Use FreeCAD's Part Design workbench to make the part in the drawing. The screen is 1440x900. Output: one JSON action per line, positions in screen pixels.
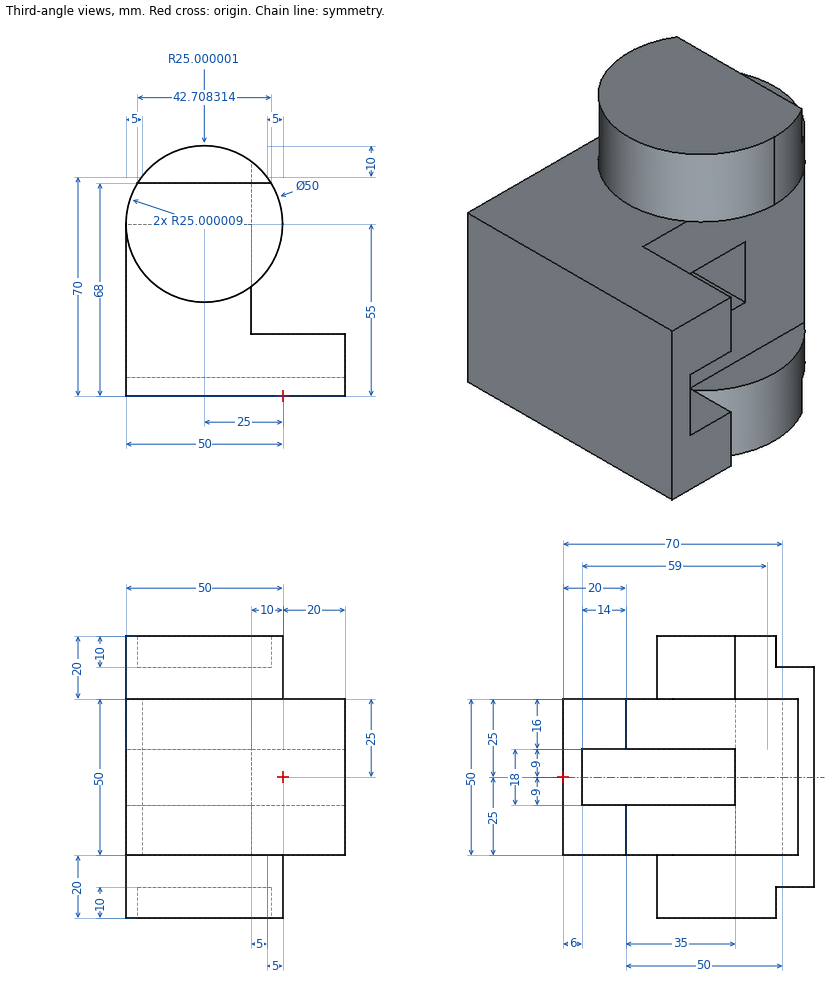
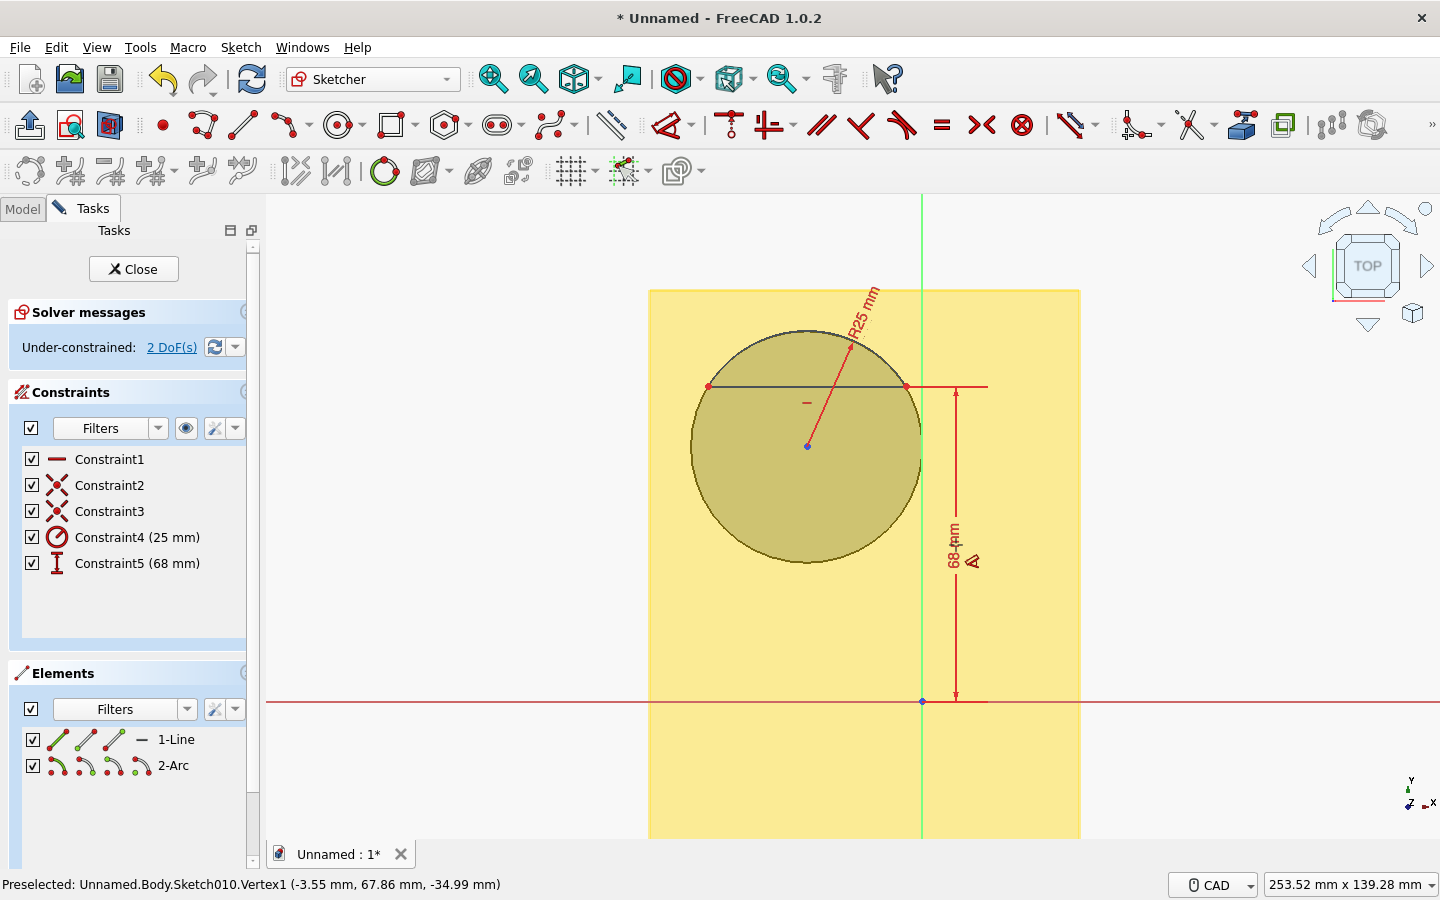
{"action": "left_click", "coordinate": [807, 447]}
{"action": "left_click", "coordinate": [865, 736]}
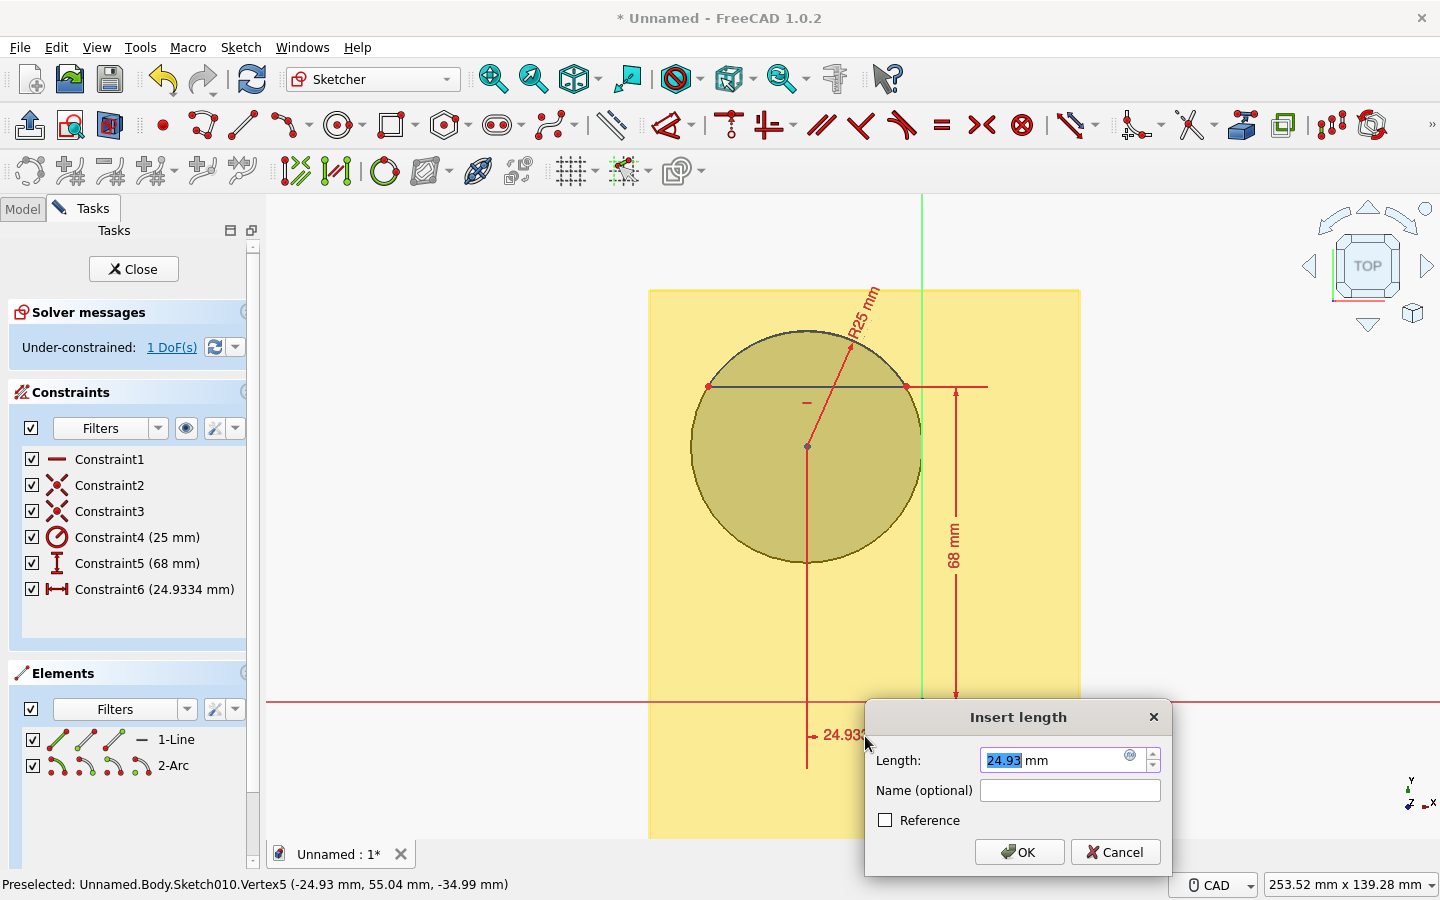
{"action": "type", "text": "25"}
{"action": "key", "text": "Return"}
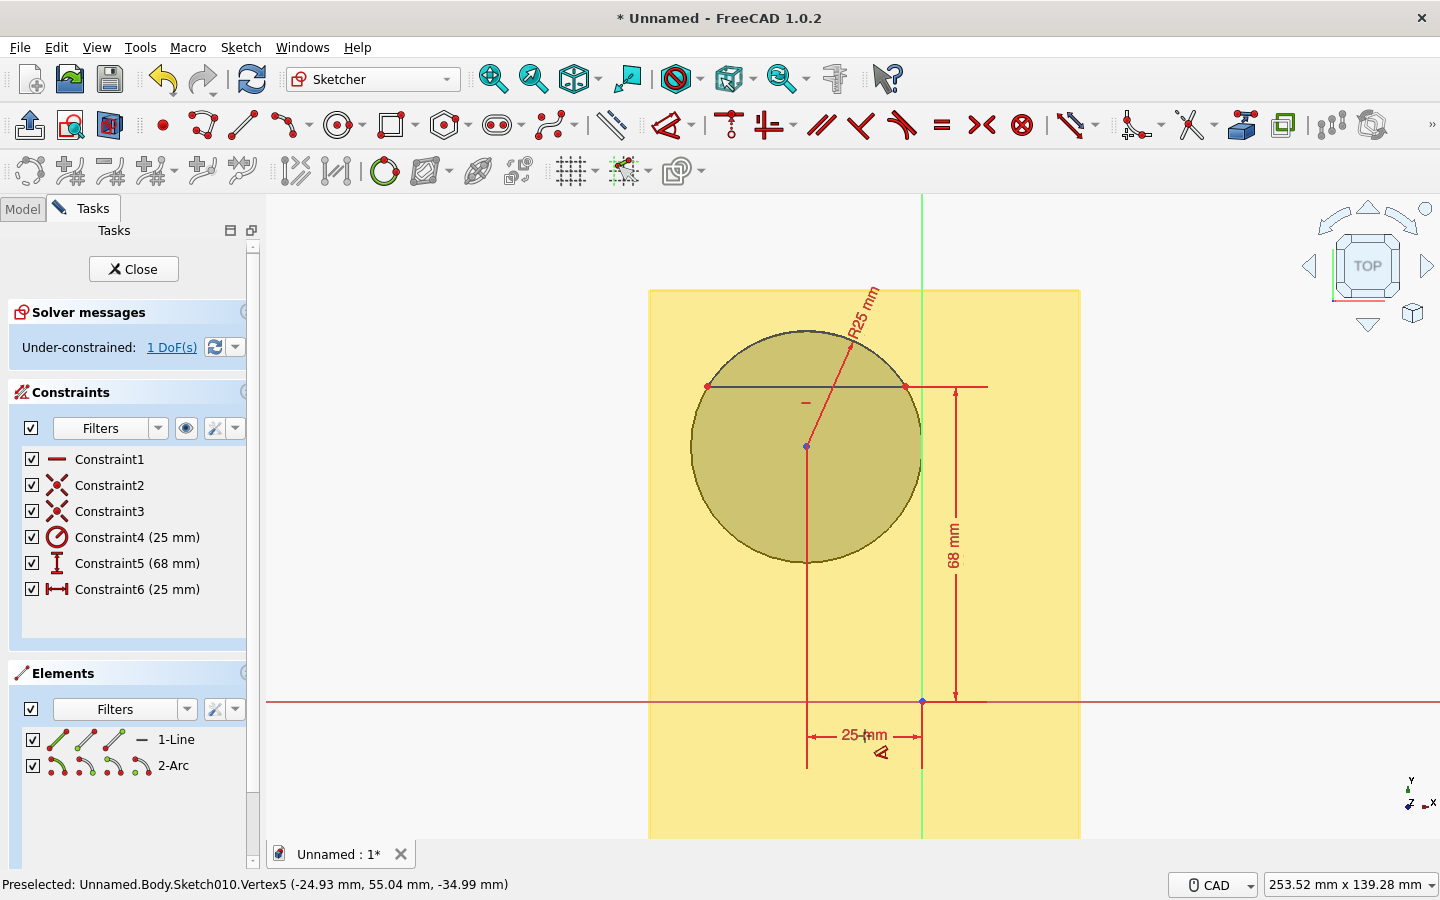
{"action": "left_click", "coordinate": [846, 387]}
{"action": "left_click", "coordinate": [807, 353]}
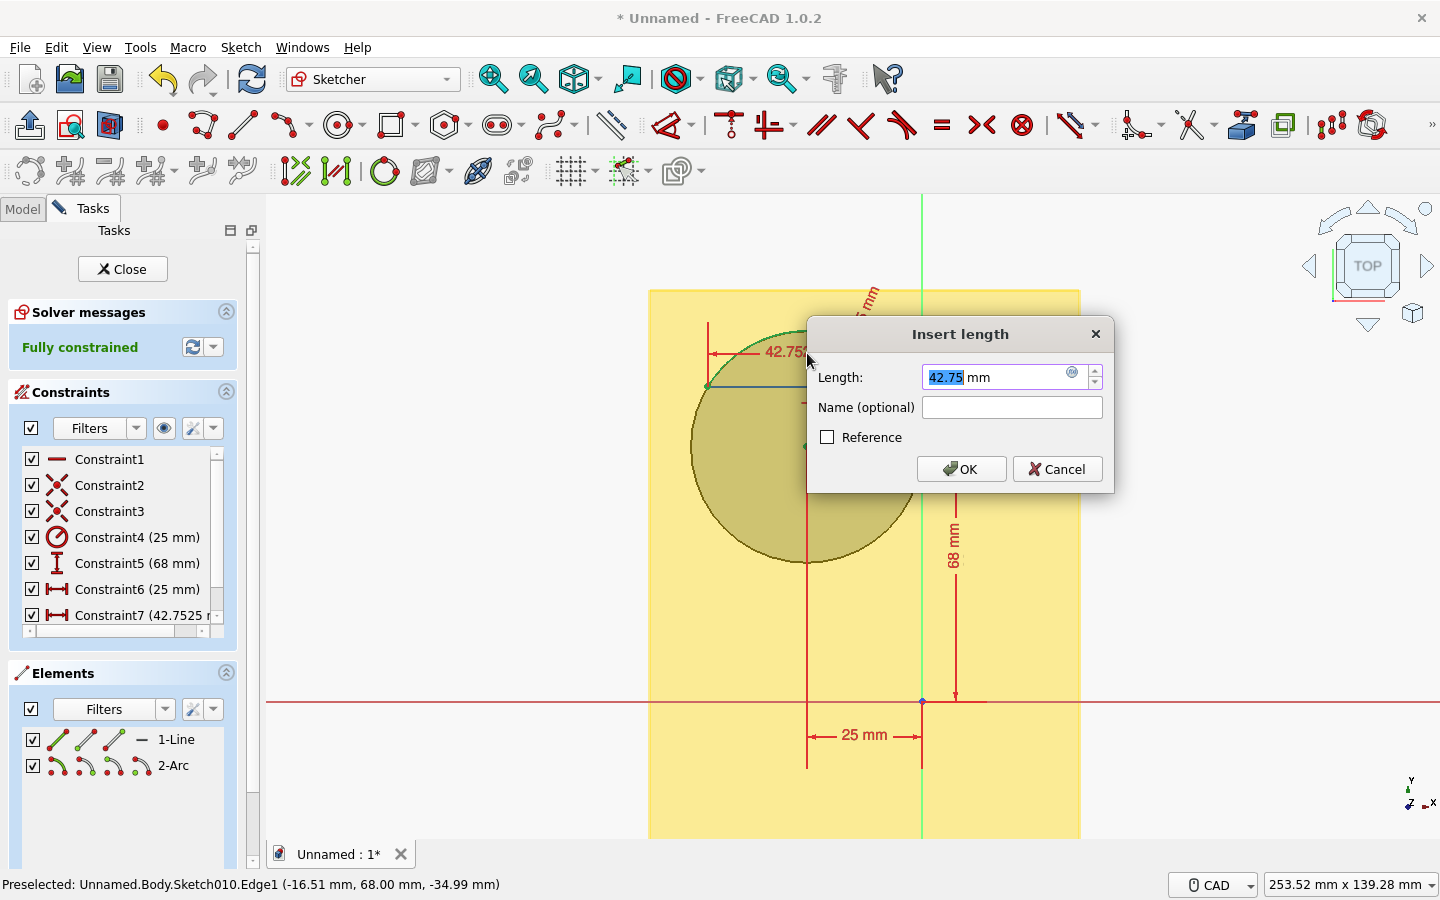
{"action": "type", "text": "42.708314"}
{"action": "key", "text": "Return"}
{"action": "key", "text": "Escape"}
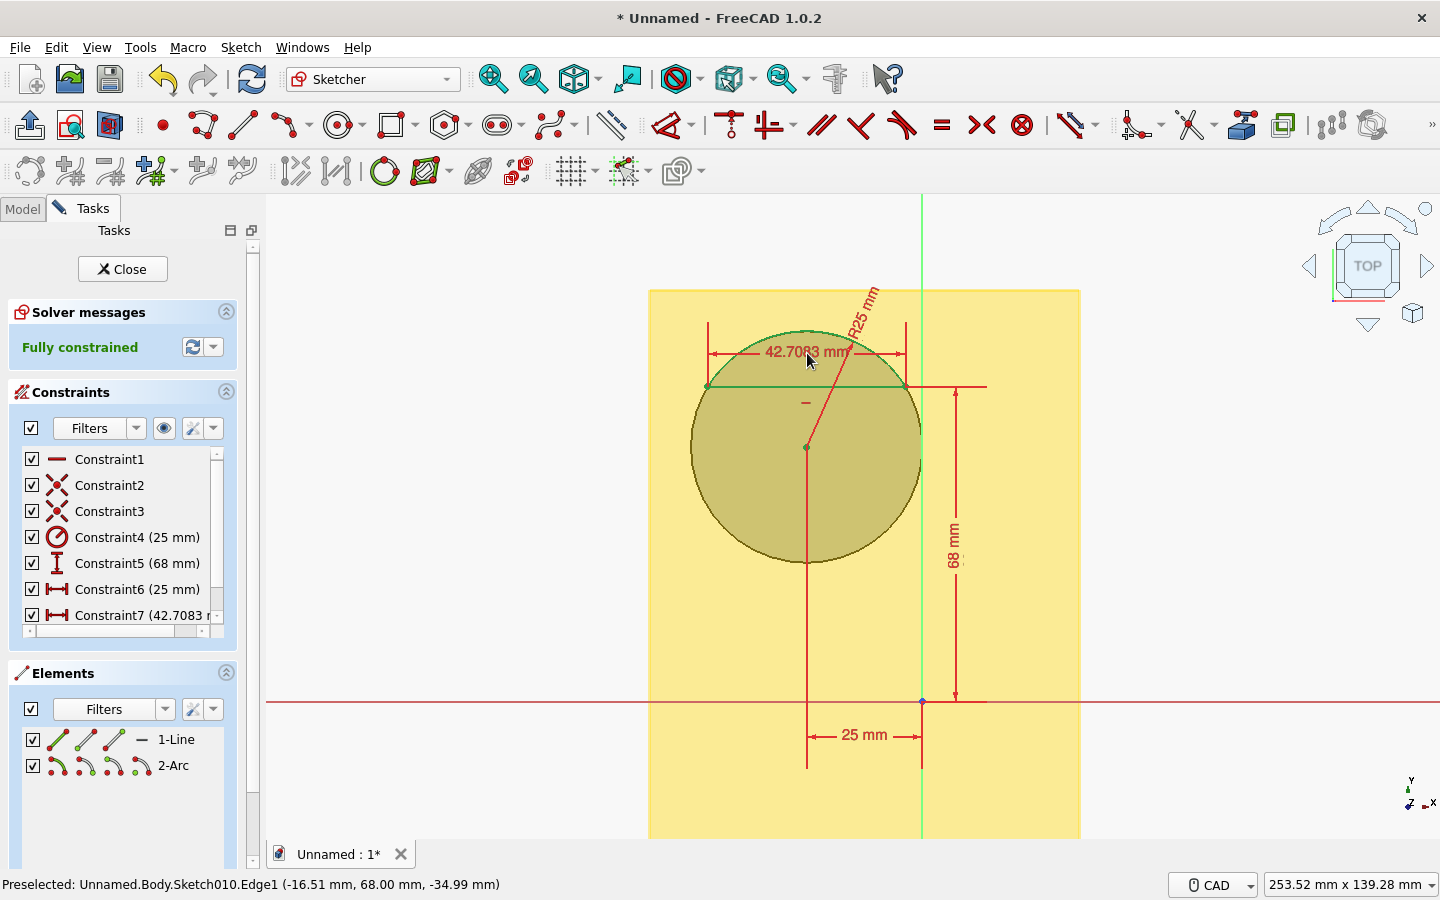
{"action": "left_click", "coordinate": [123, 269]}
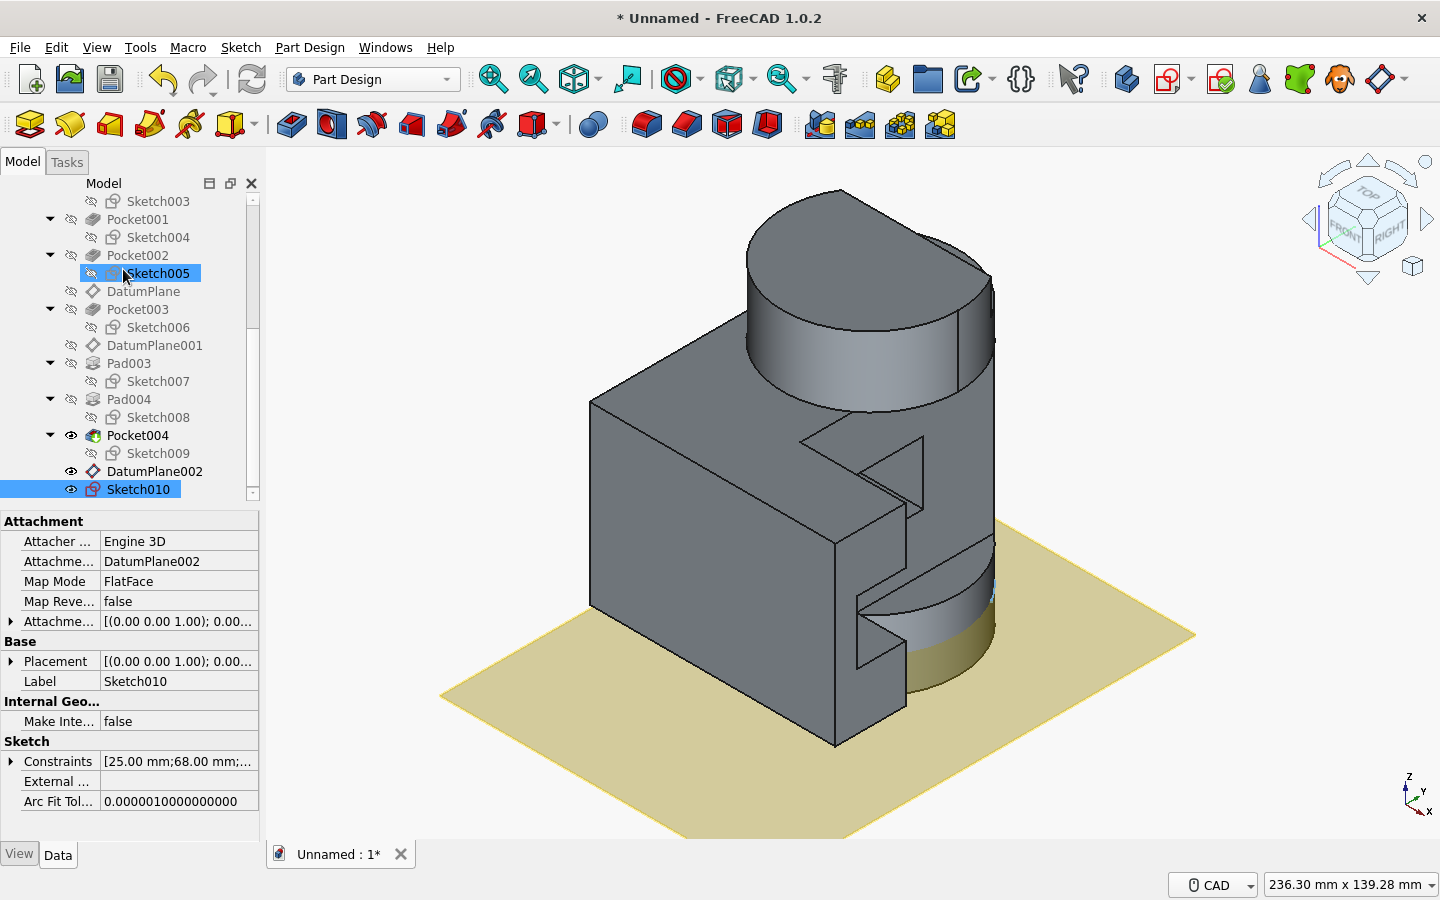
{"action": "left_click", "coordinate": [292, 124]}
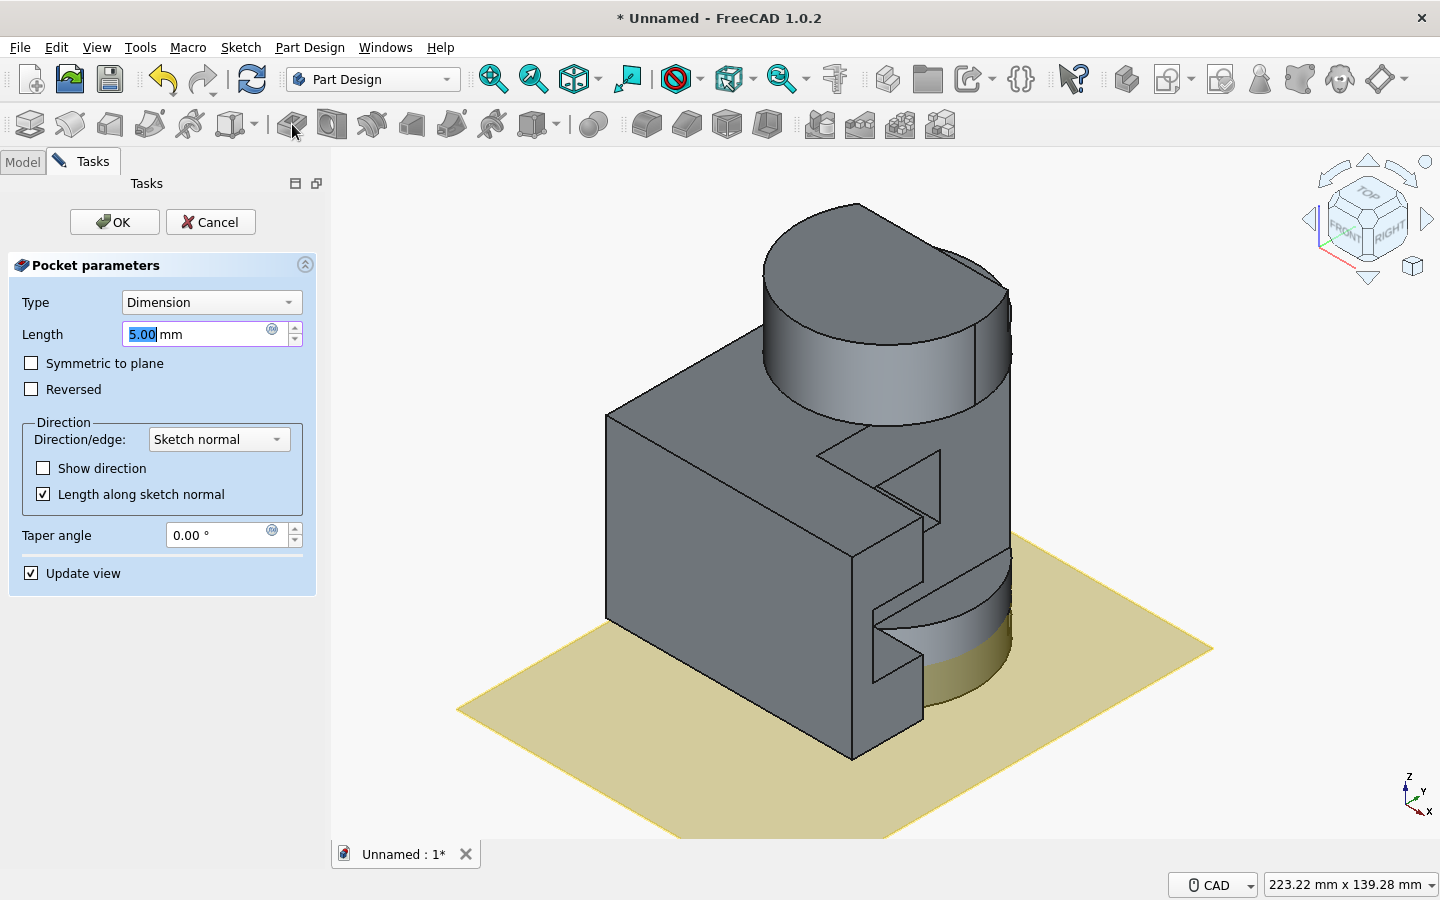
{"action": "type", "text": "10"}
{"action": "key", "text": "Tab"}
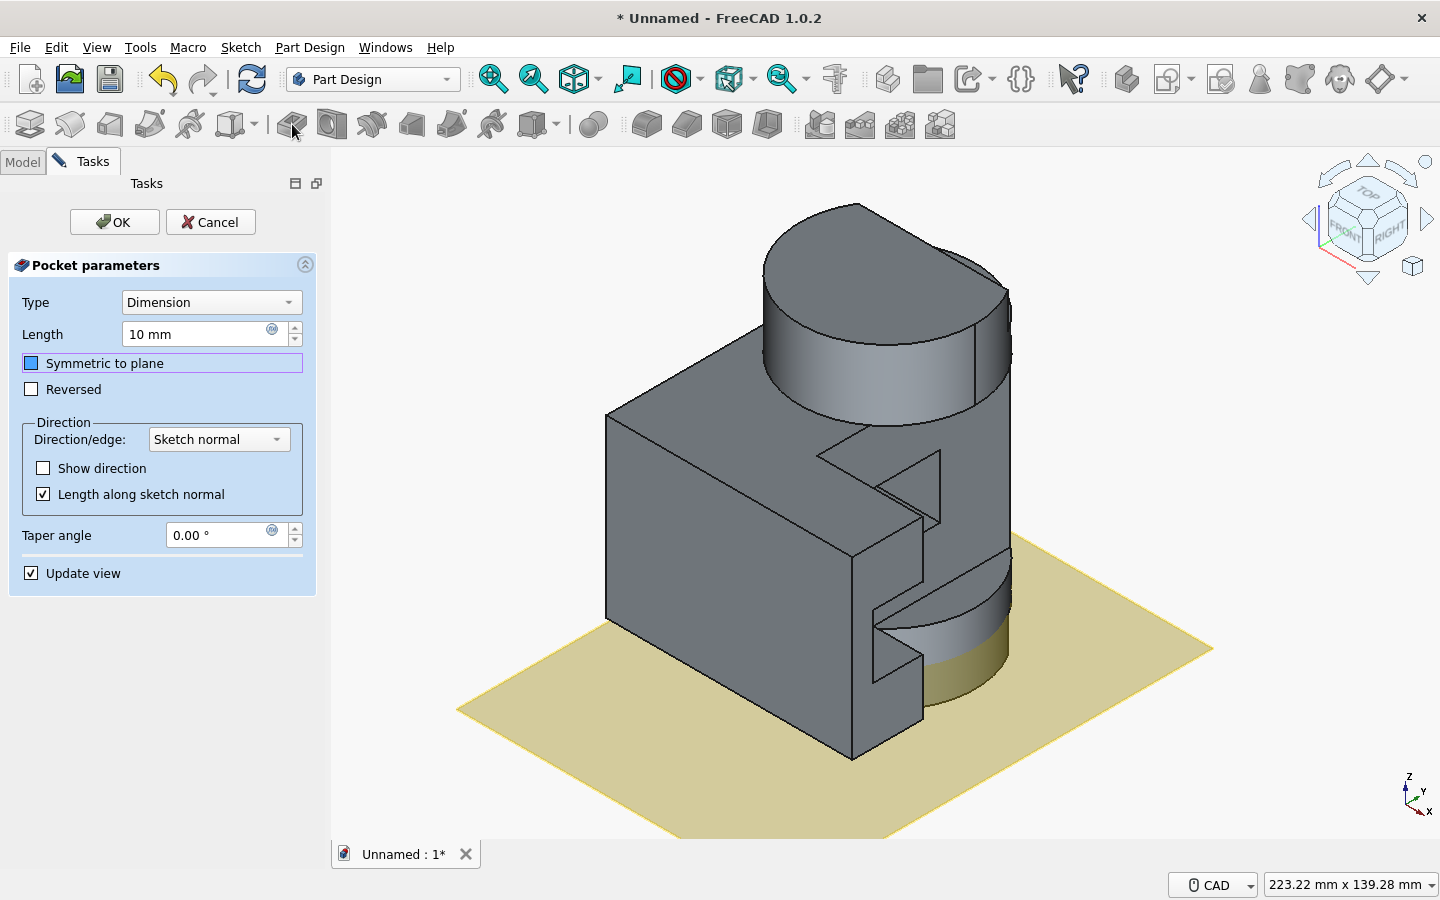
{"action": "left_click", "coordinate": [115, 222]}